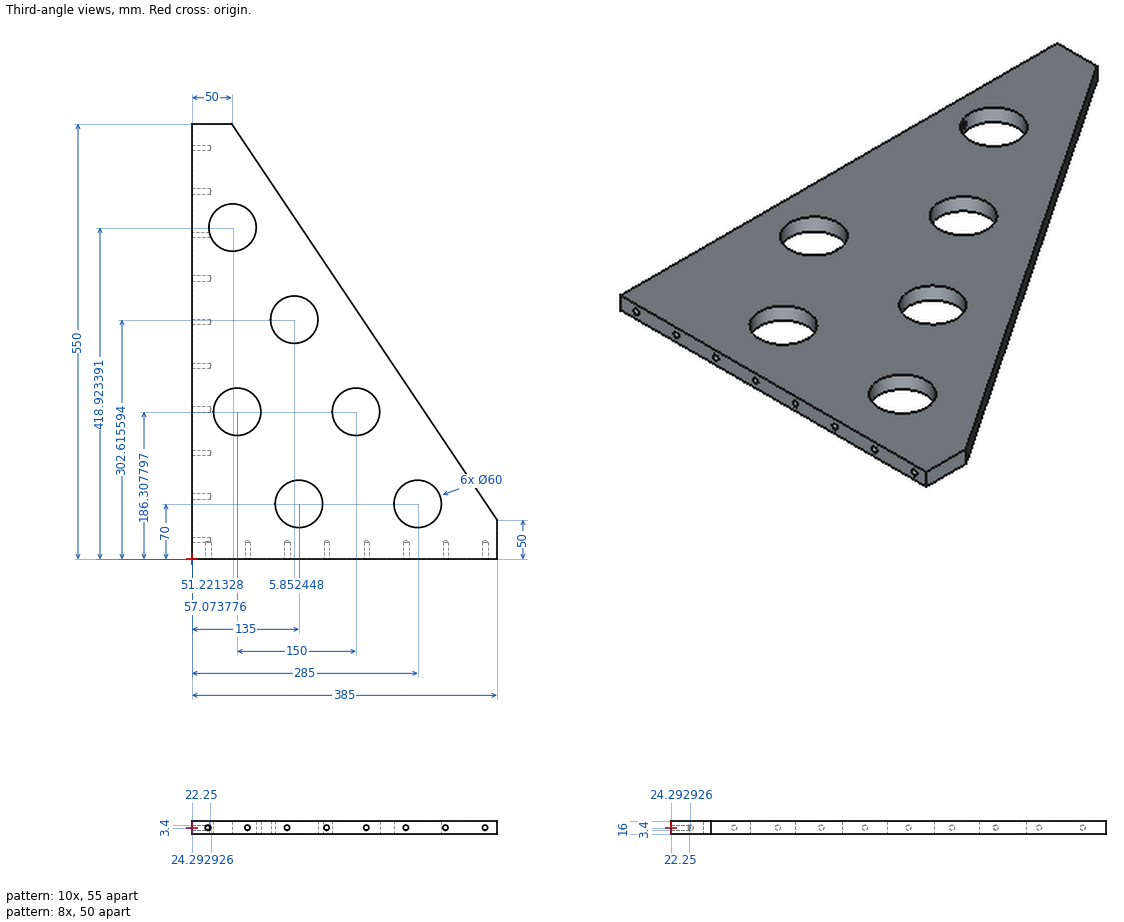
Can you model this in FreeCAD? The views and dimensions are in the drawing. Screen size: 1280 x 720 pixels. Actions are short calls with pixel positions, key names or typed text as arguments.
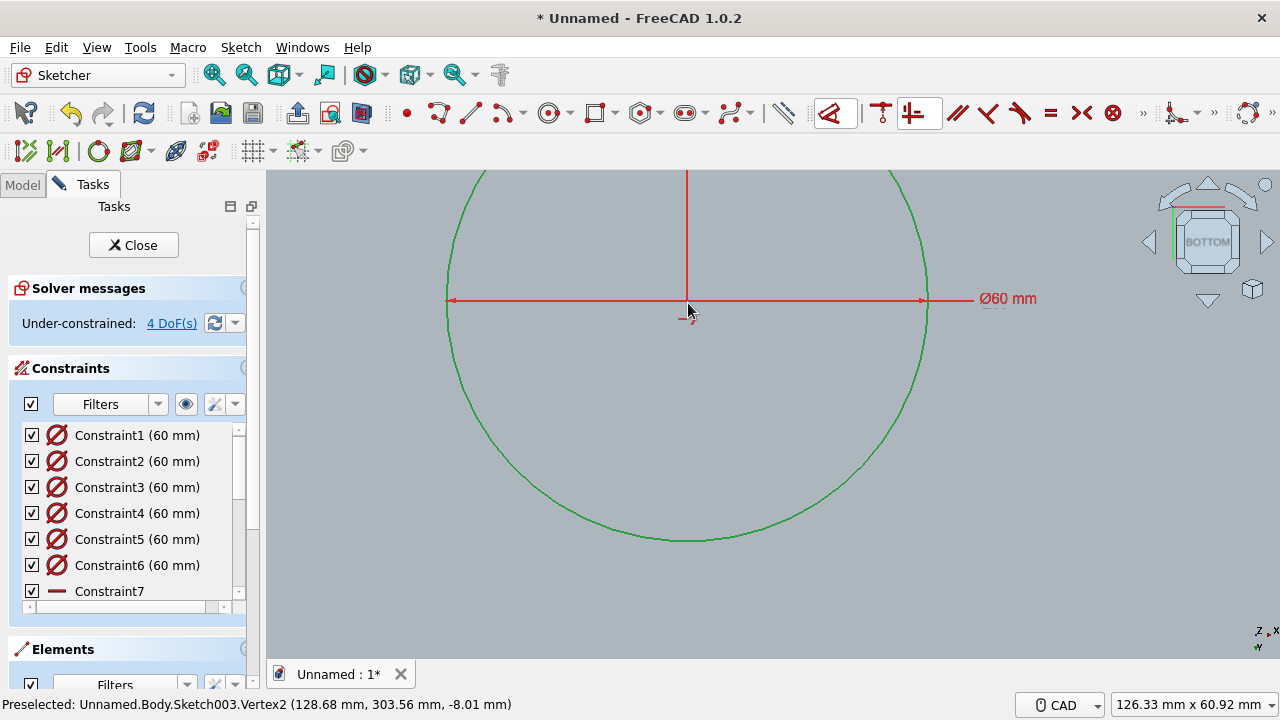
click(687, 301)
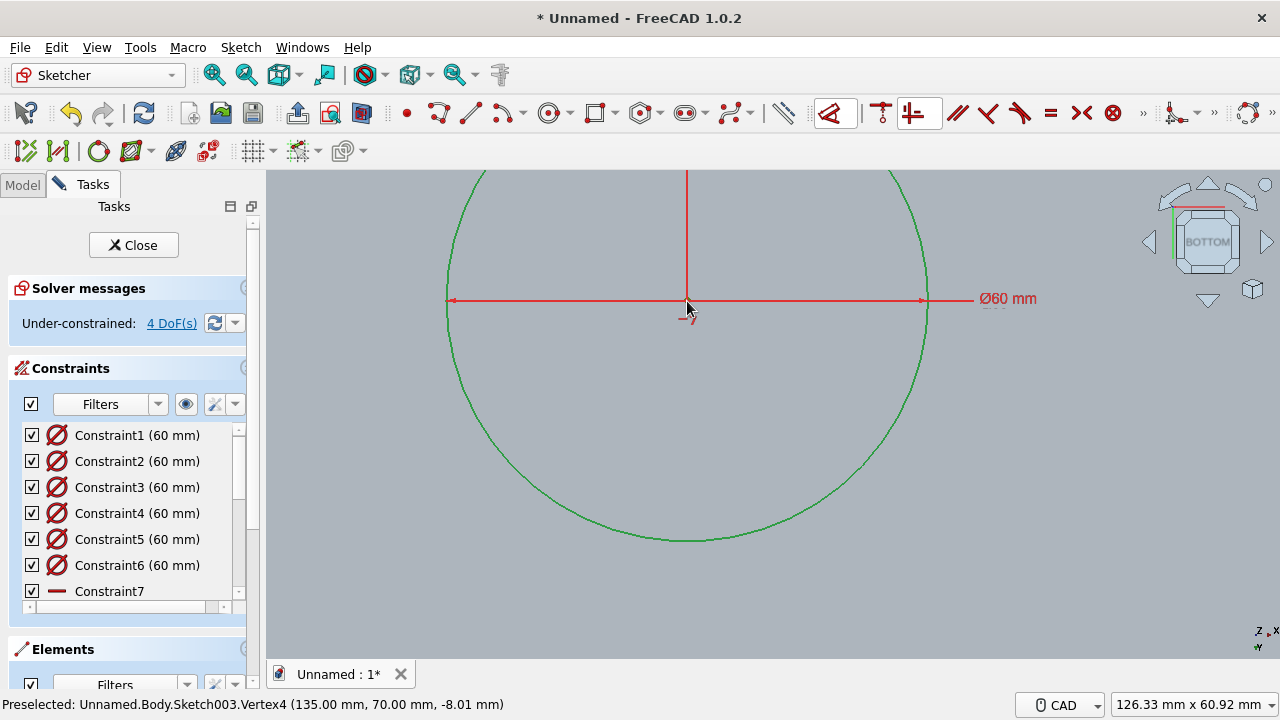
click(852, 114)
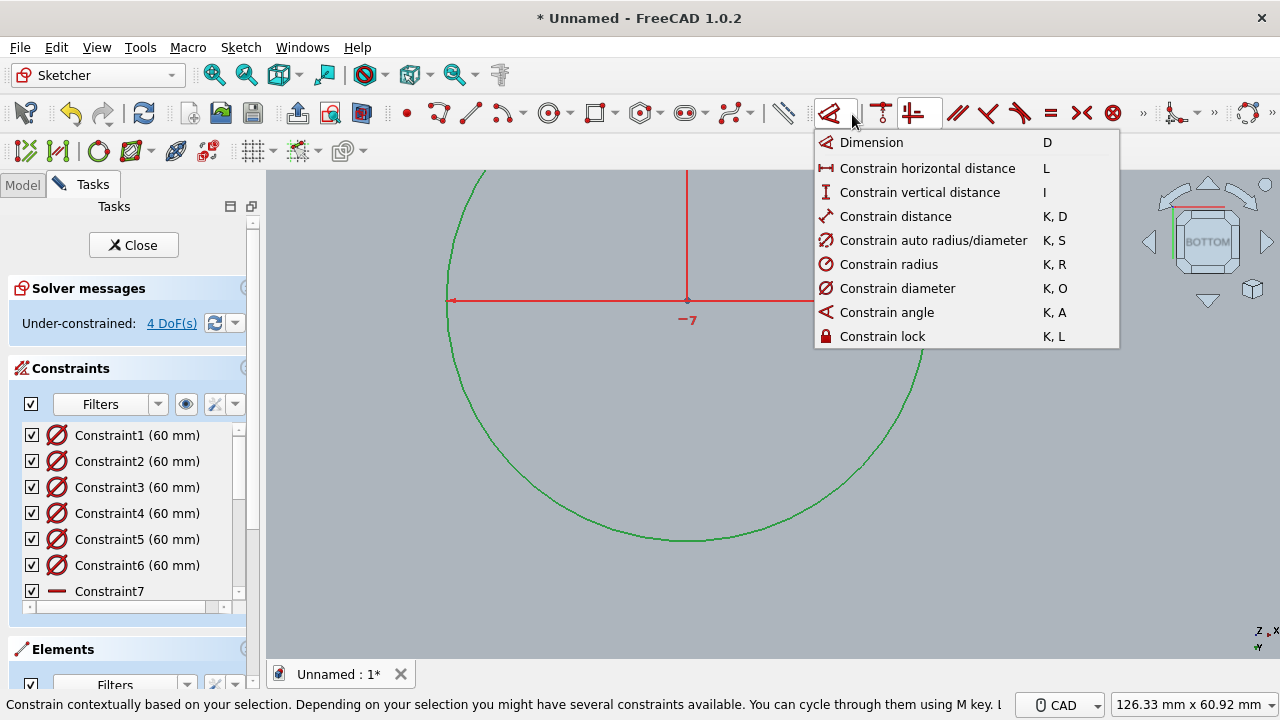
click(967, 168)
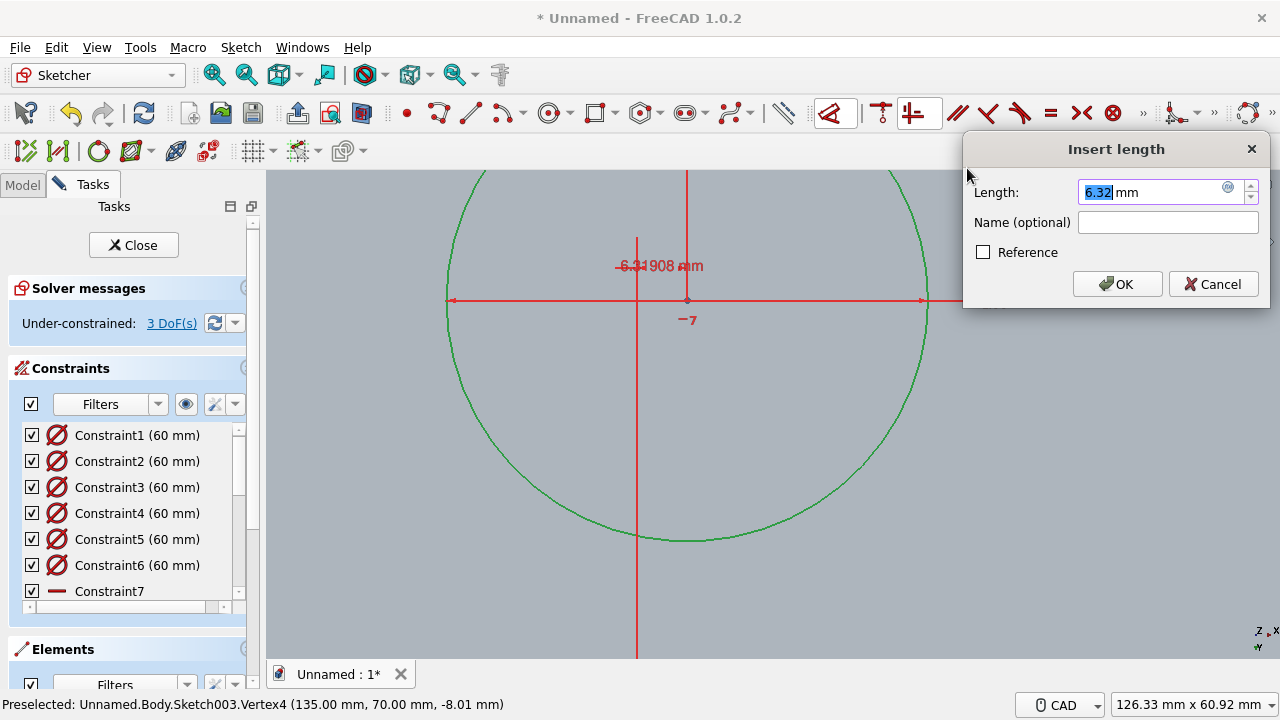
text(5.852448)
key(Return)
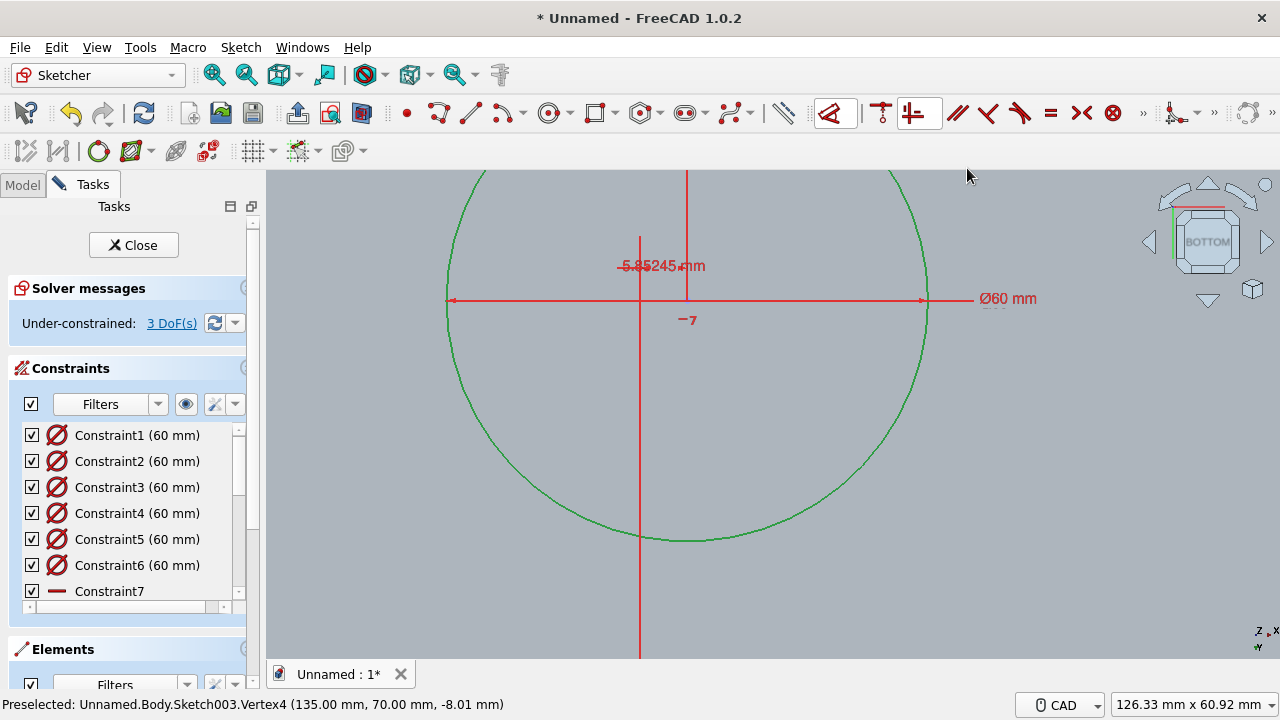
scroll(688, 302, down, 12)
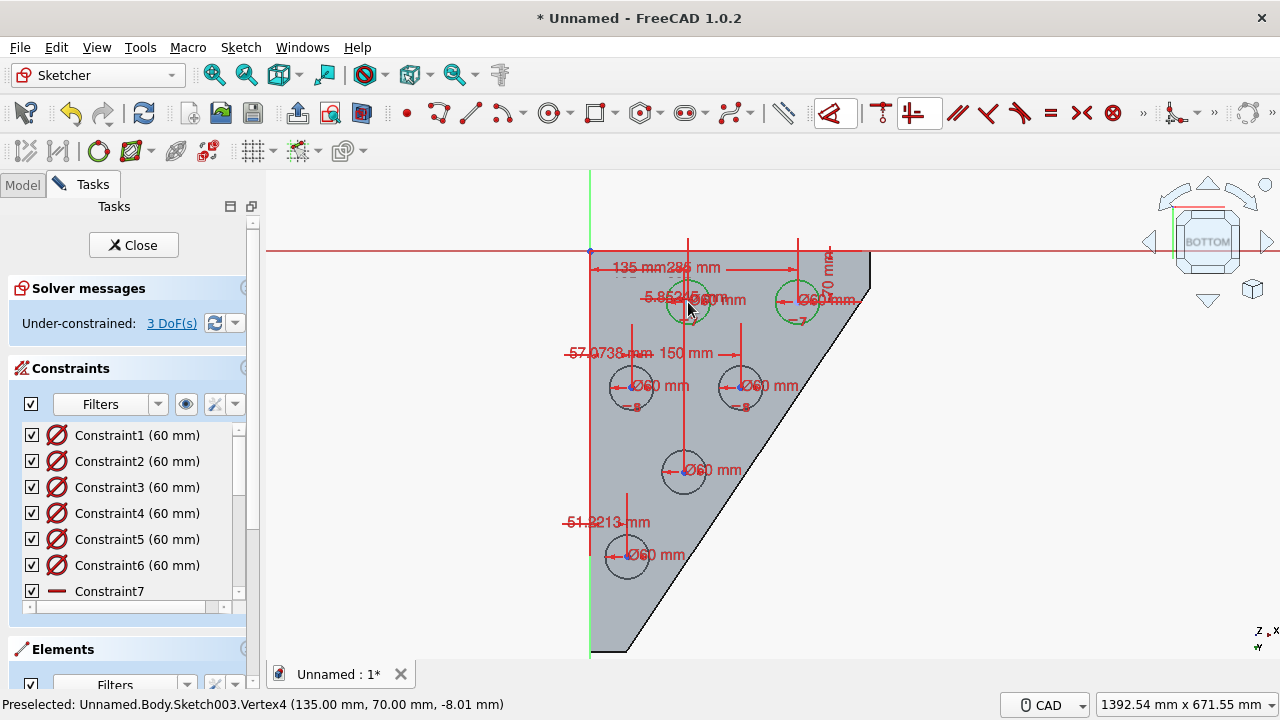
click(684, 472)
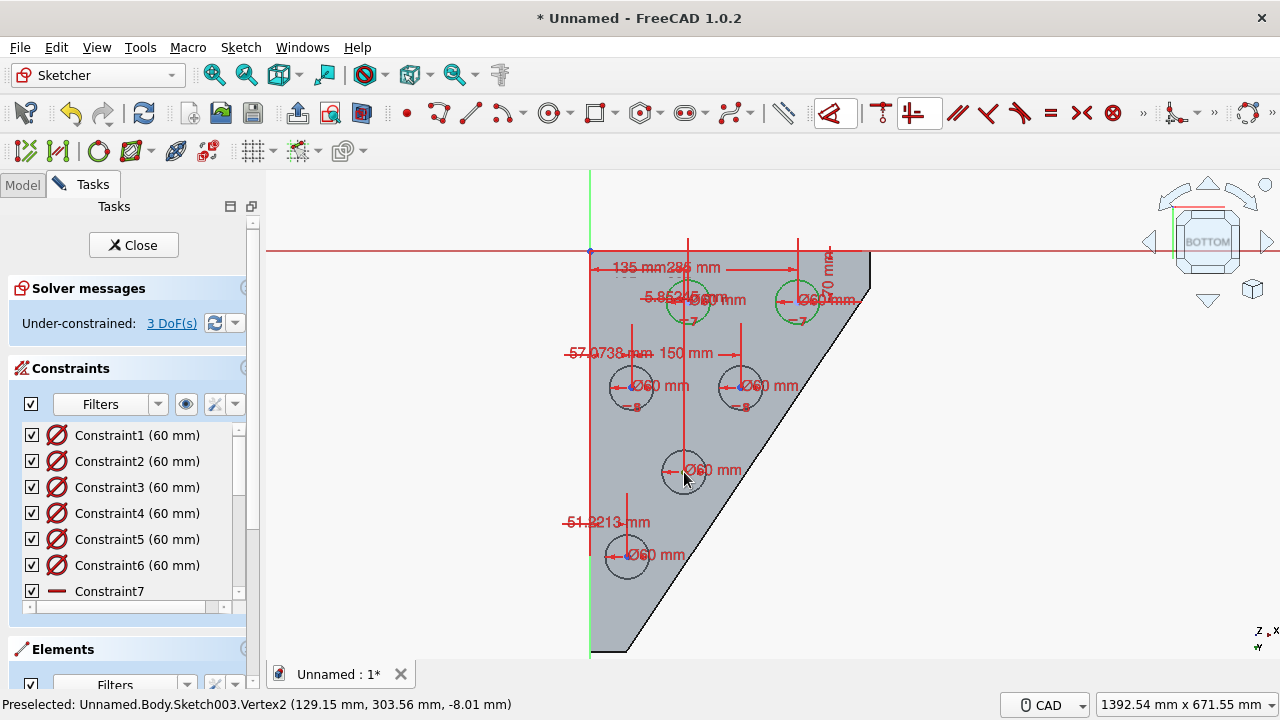
key(i)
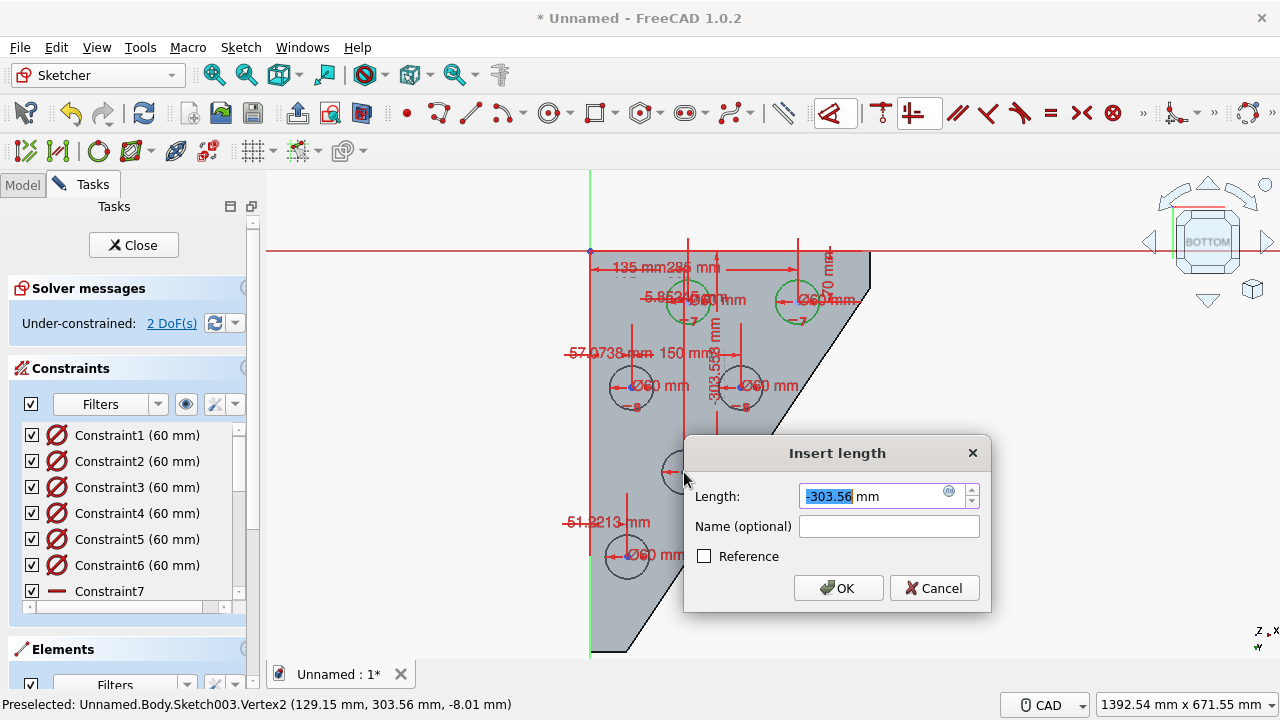
text(-302.615594)
key(Return)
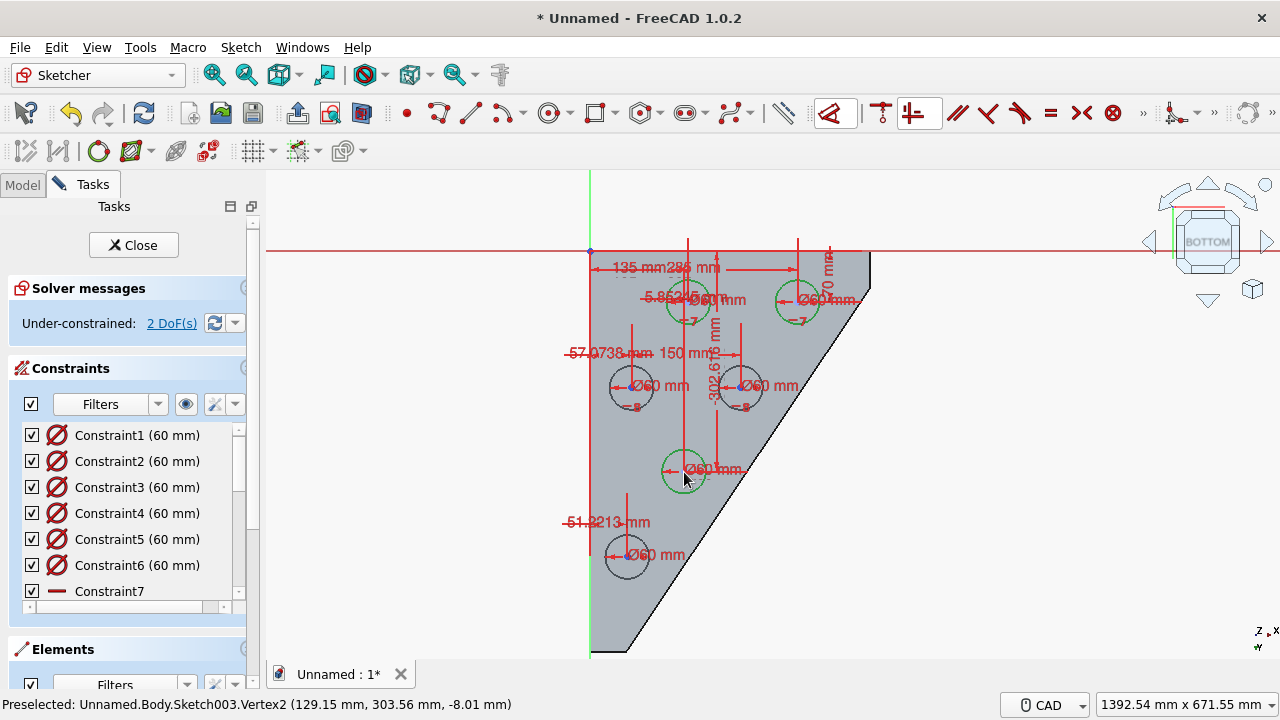
click(741, 388)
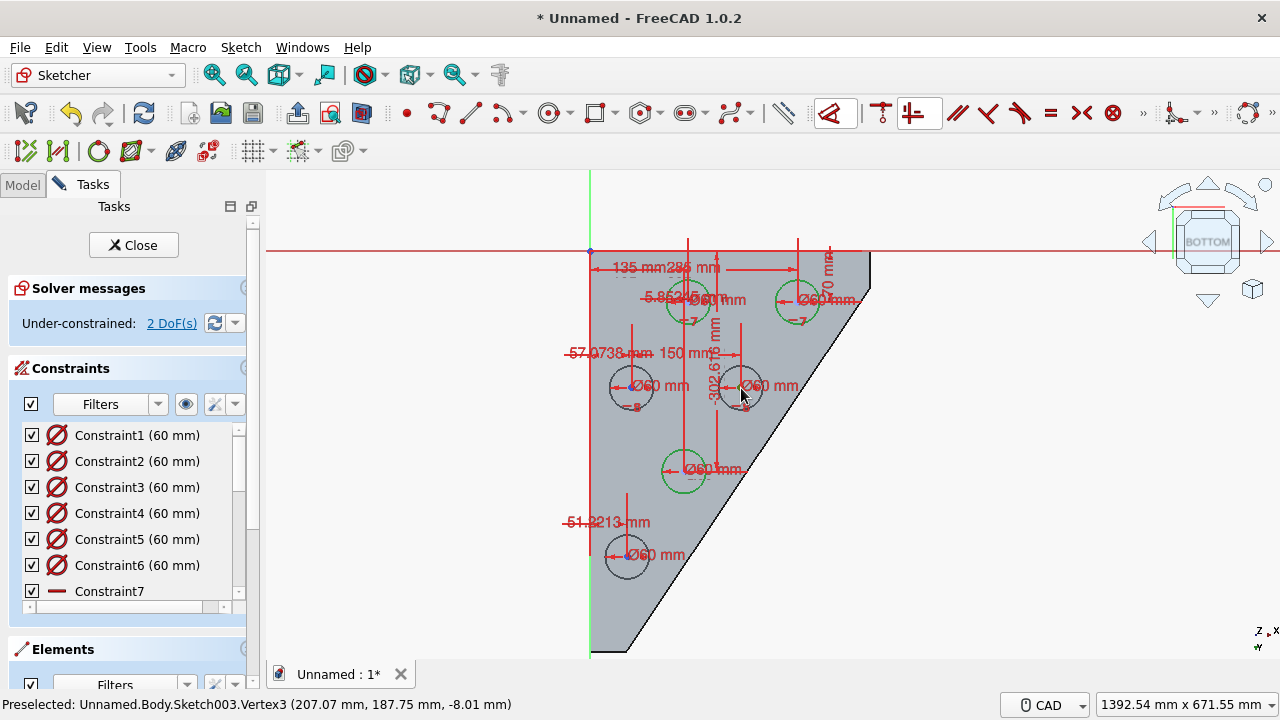
key(i)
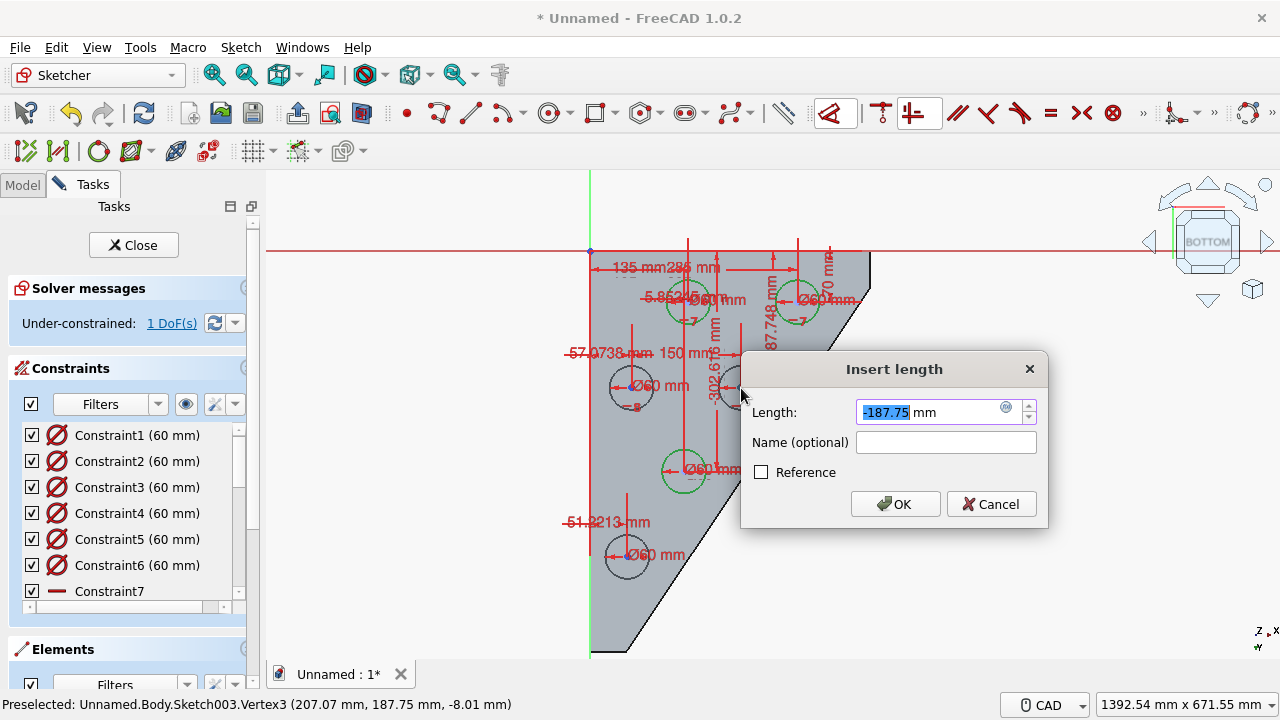
text(-186.307797)
key(Return)